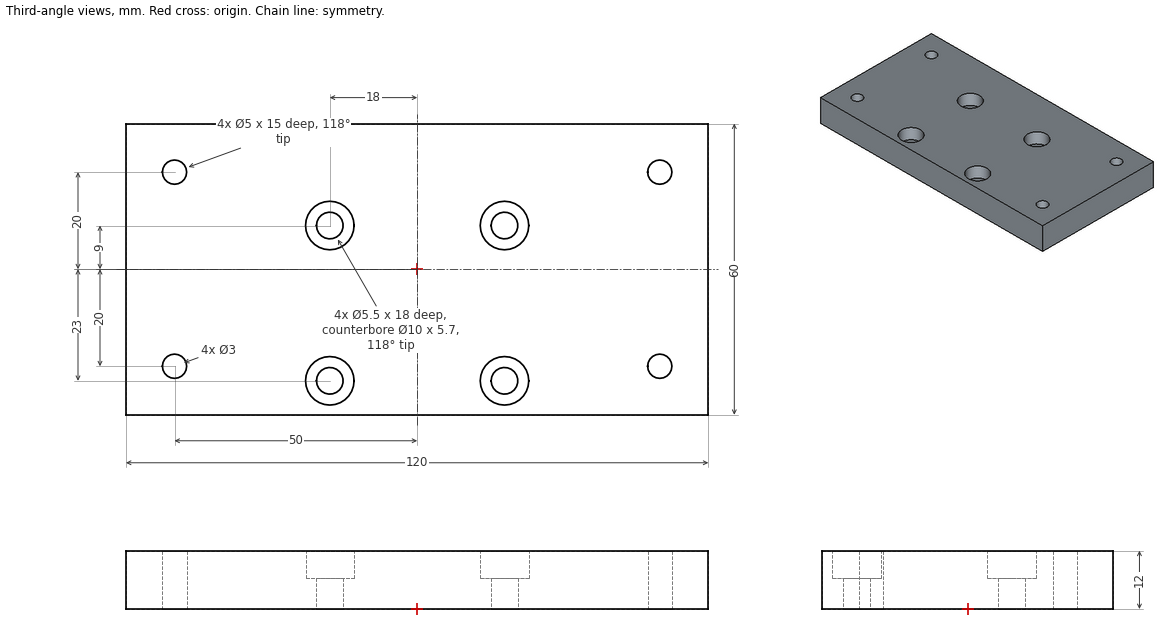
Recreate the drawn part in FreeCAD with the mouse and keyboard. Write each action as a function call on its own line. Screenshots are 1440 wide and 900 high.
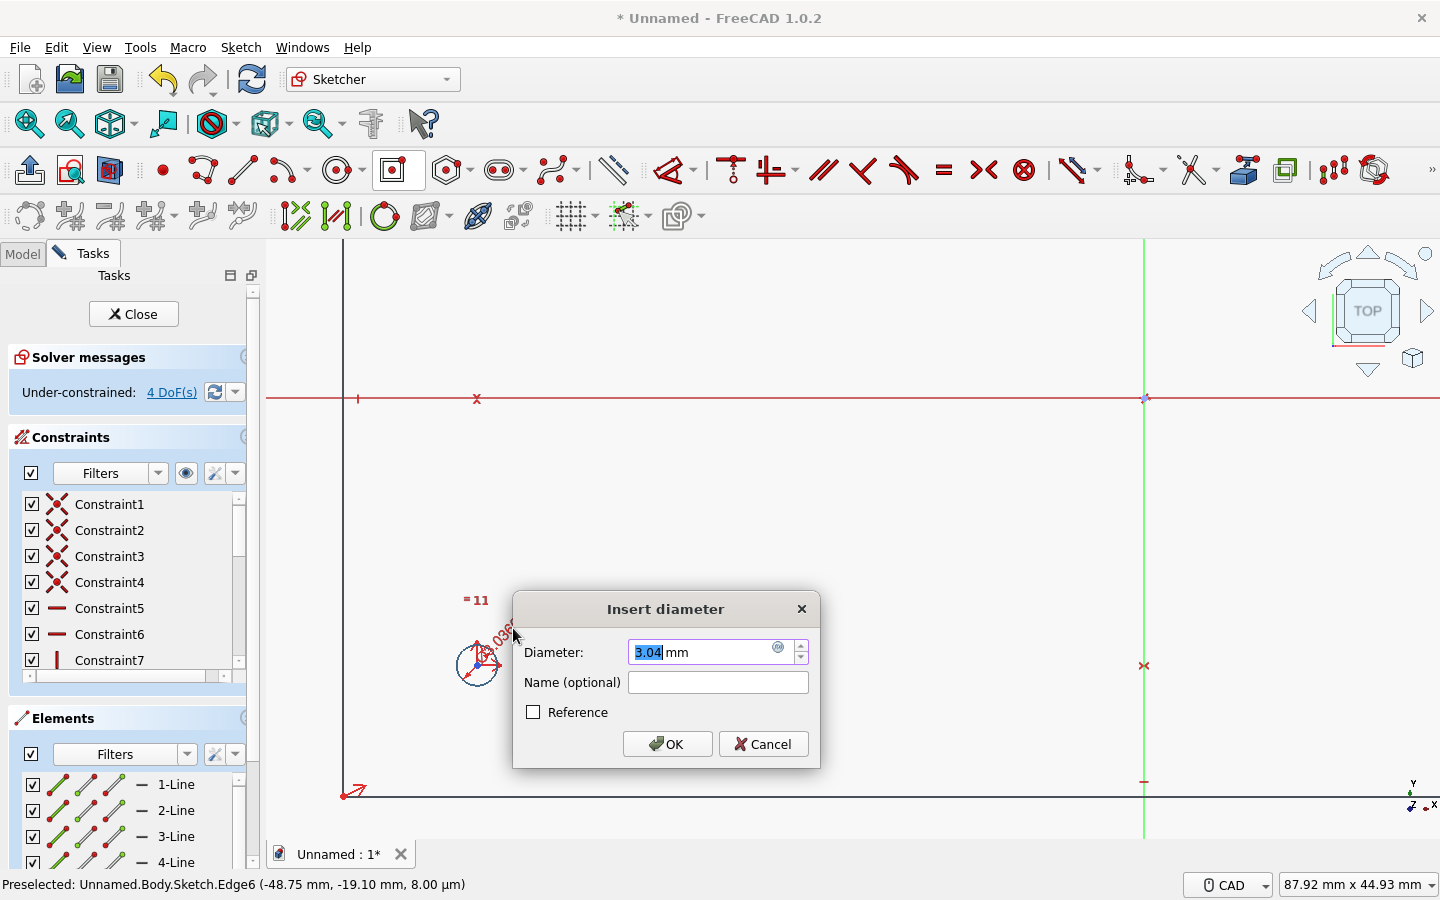
text(3)
key(Return)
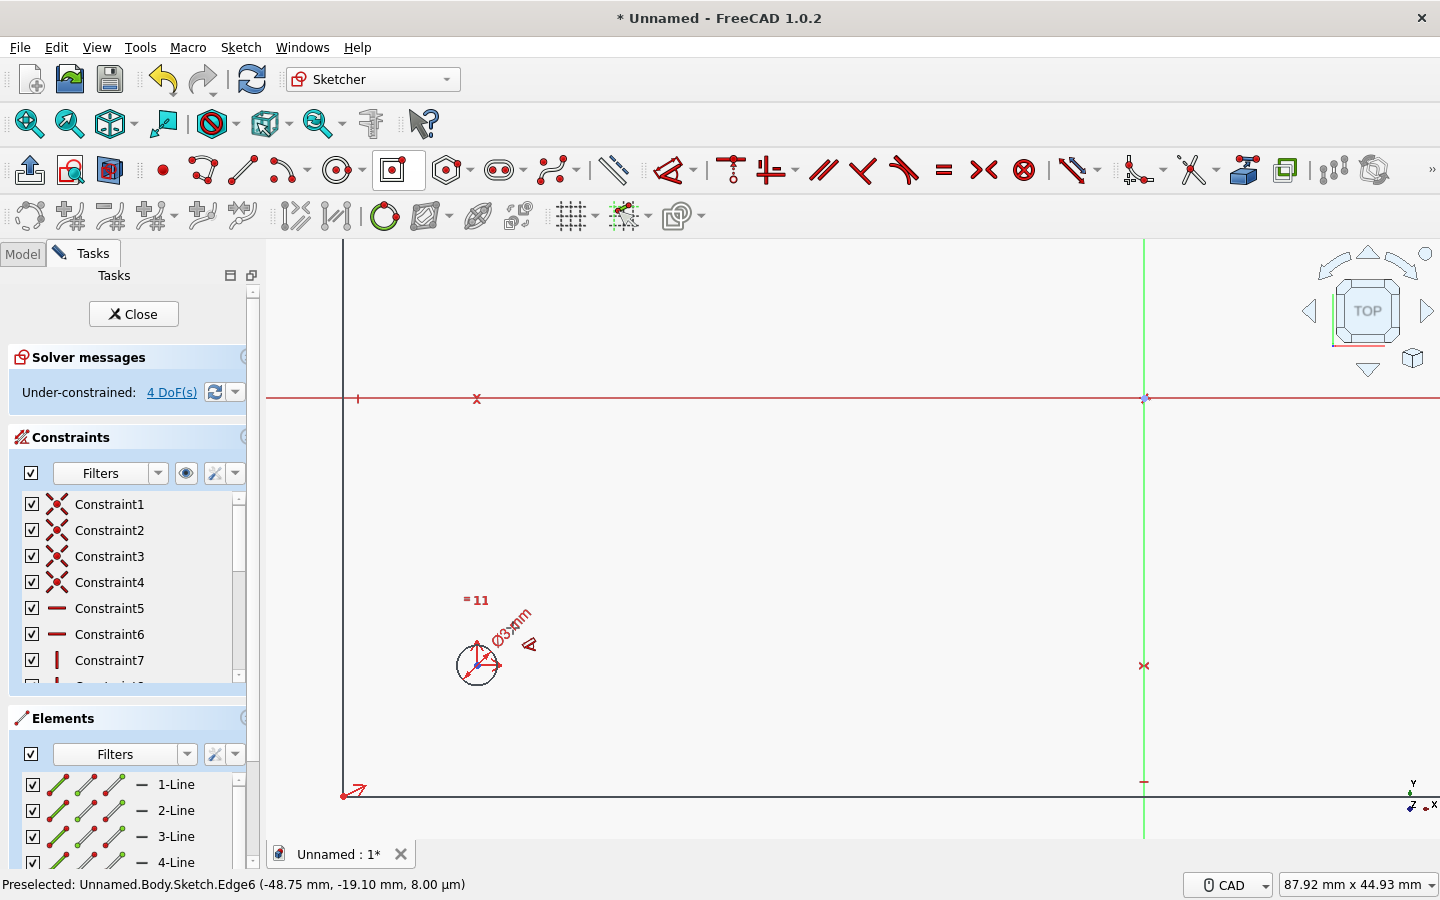
scroll(491, 654, down, 4)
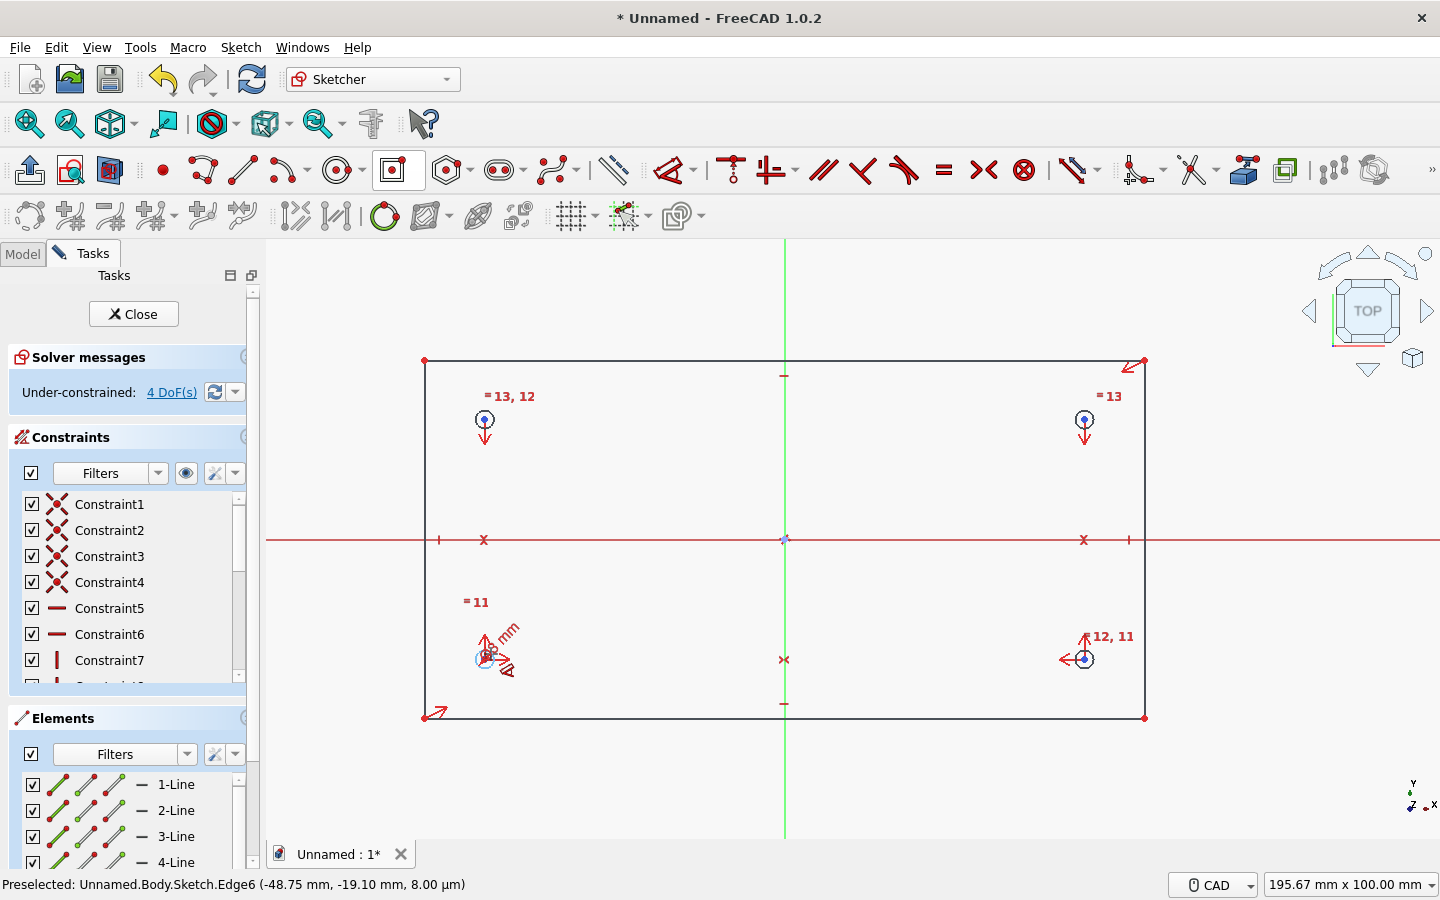
click(1145, 611)
click(1179, 457)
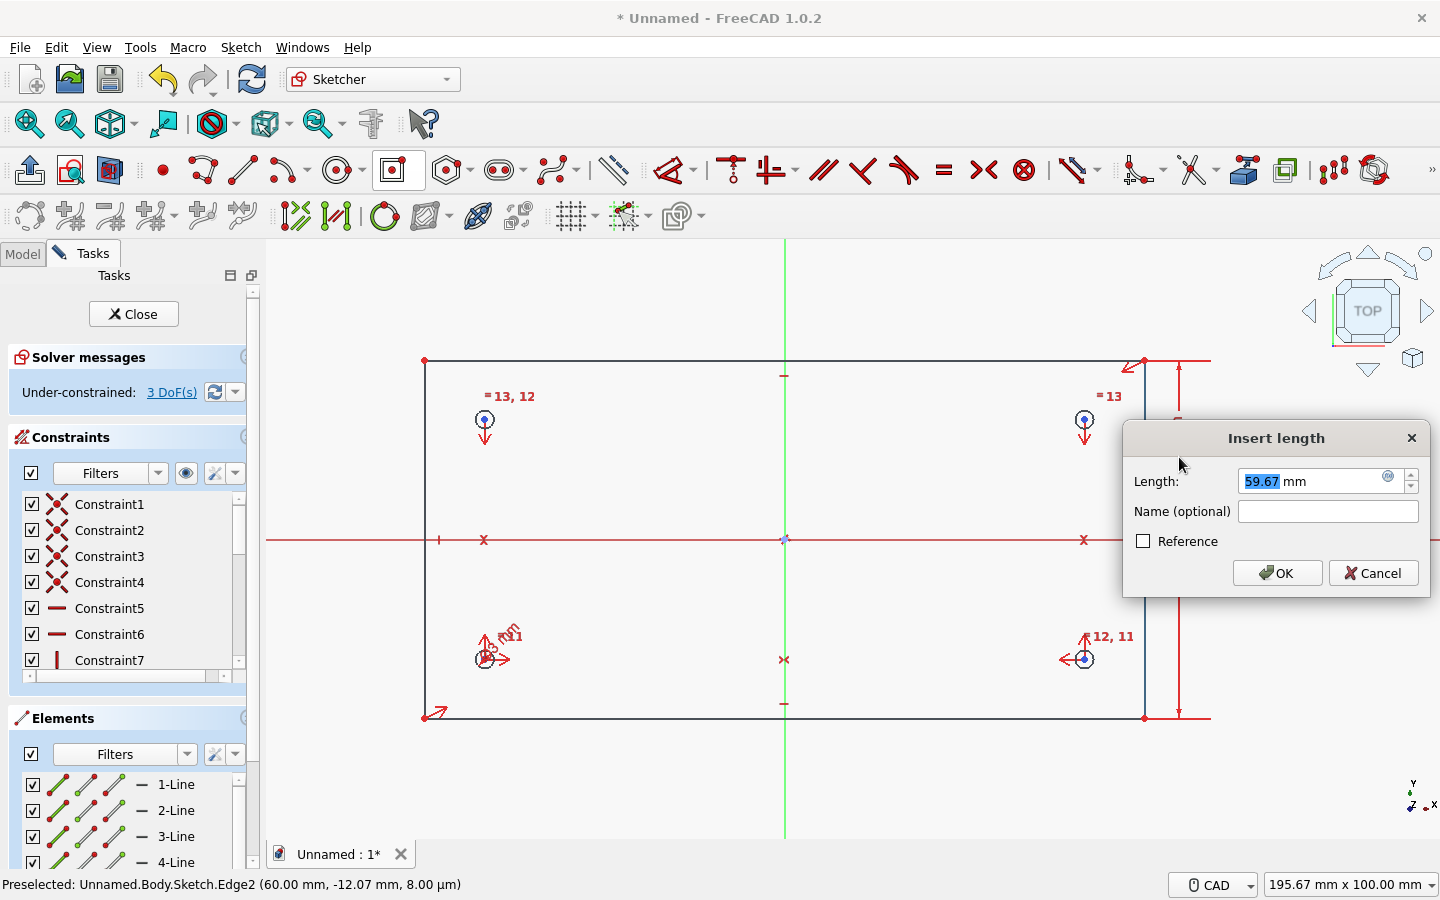
text(60)
key(Return)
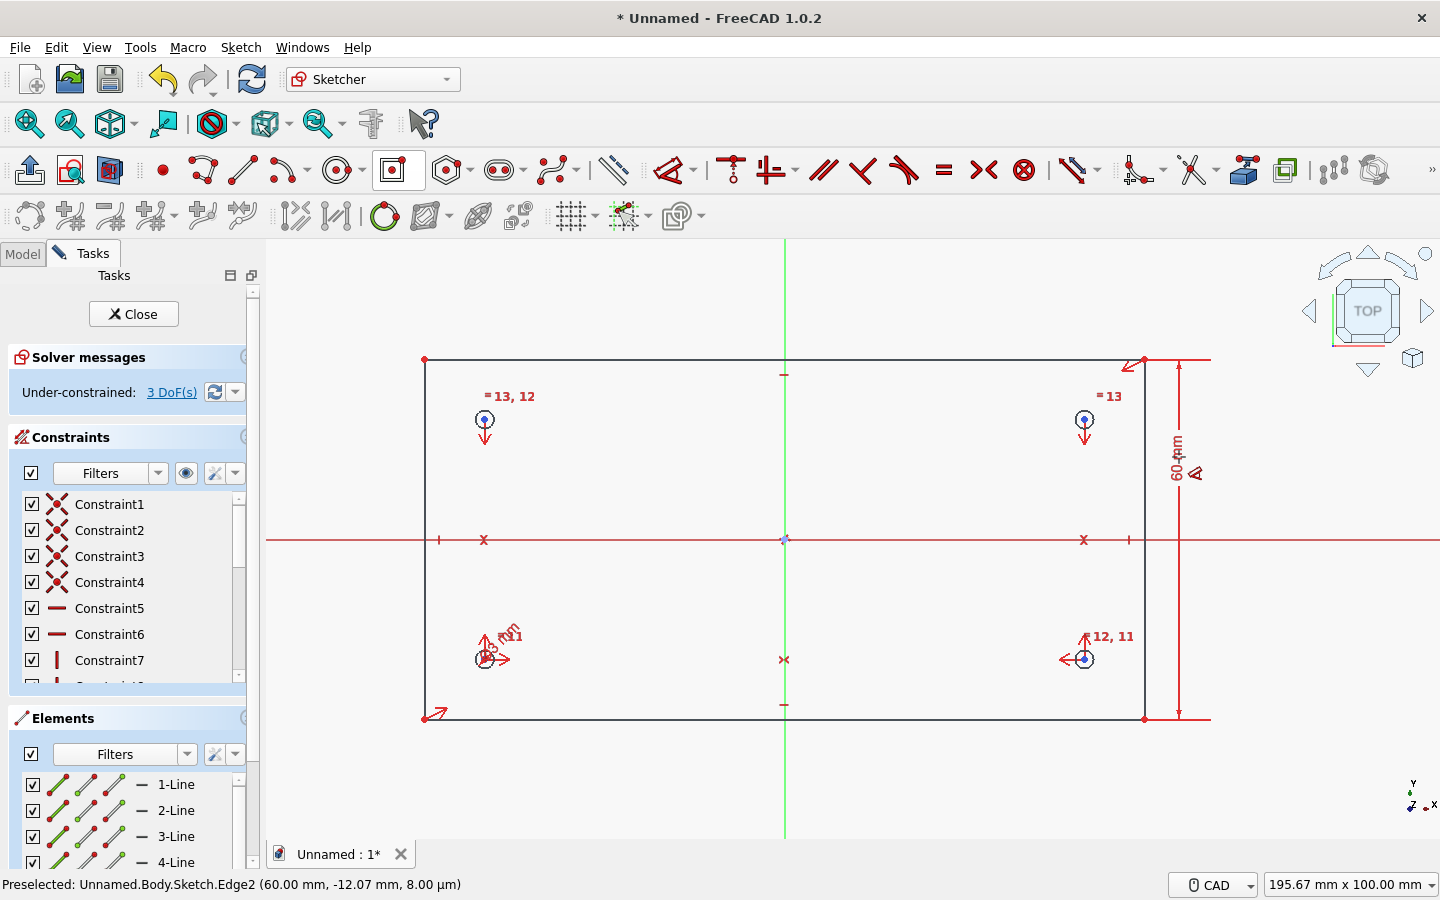
click(485, 660)
click(635, 694)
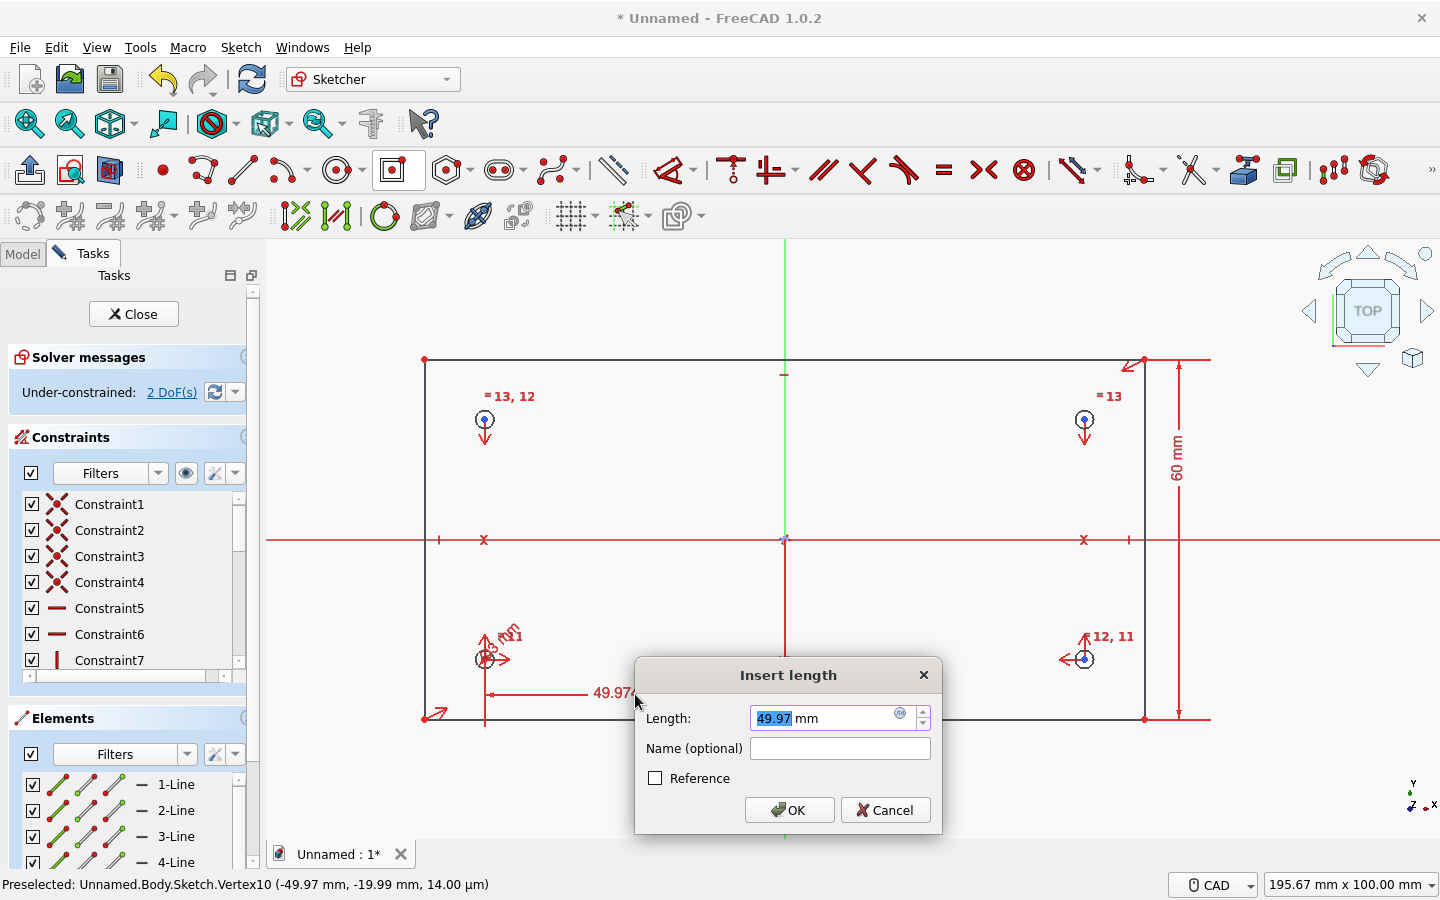
text(50)
key(Return)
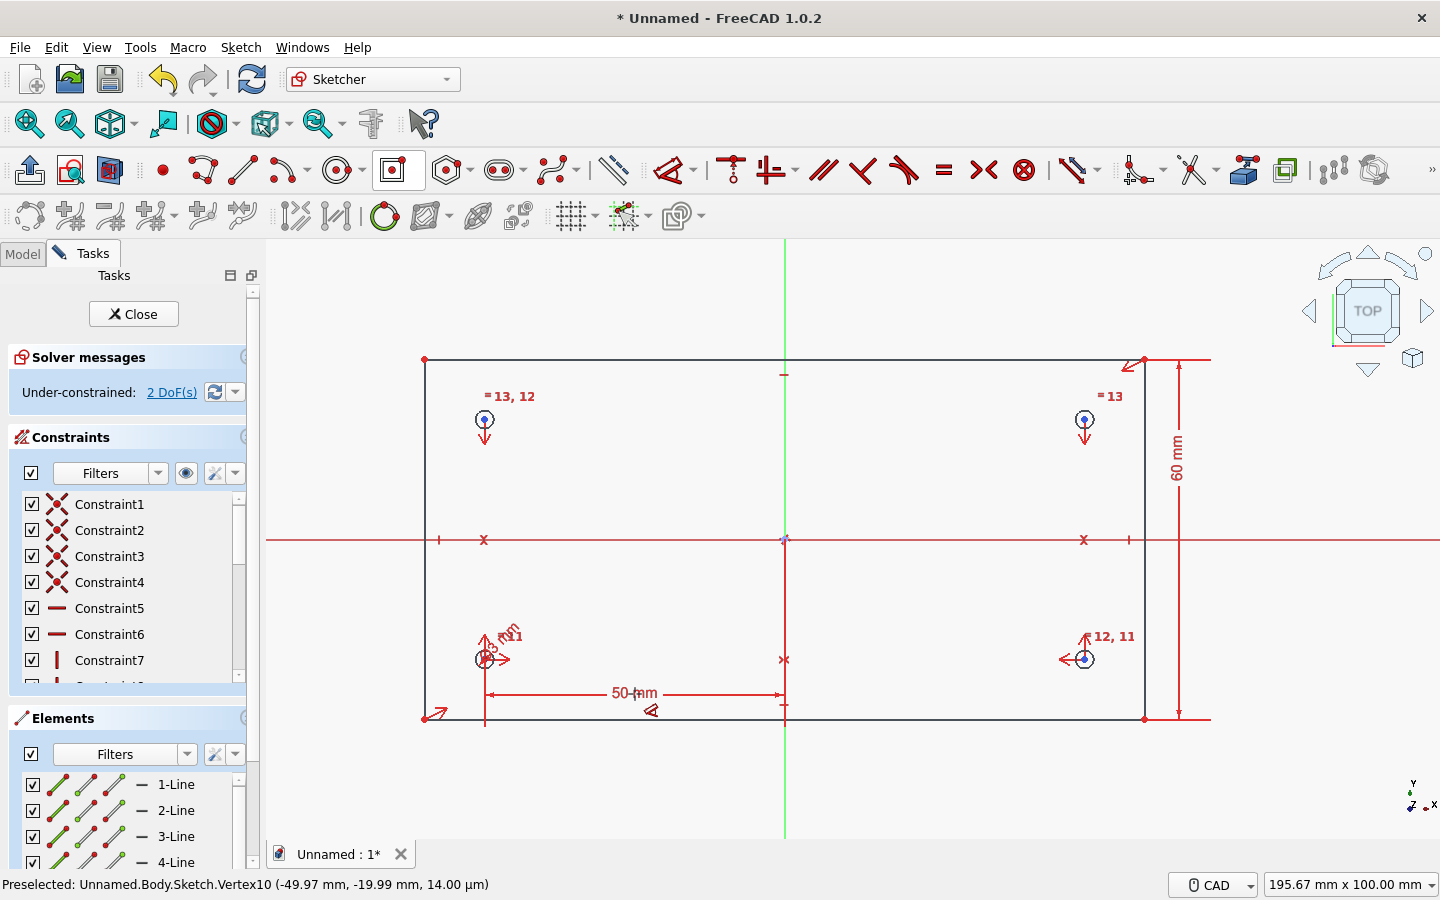
click(485, 660)
click(451, 600)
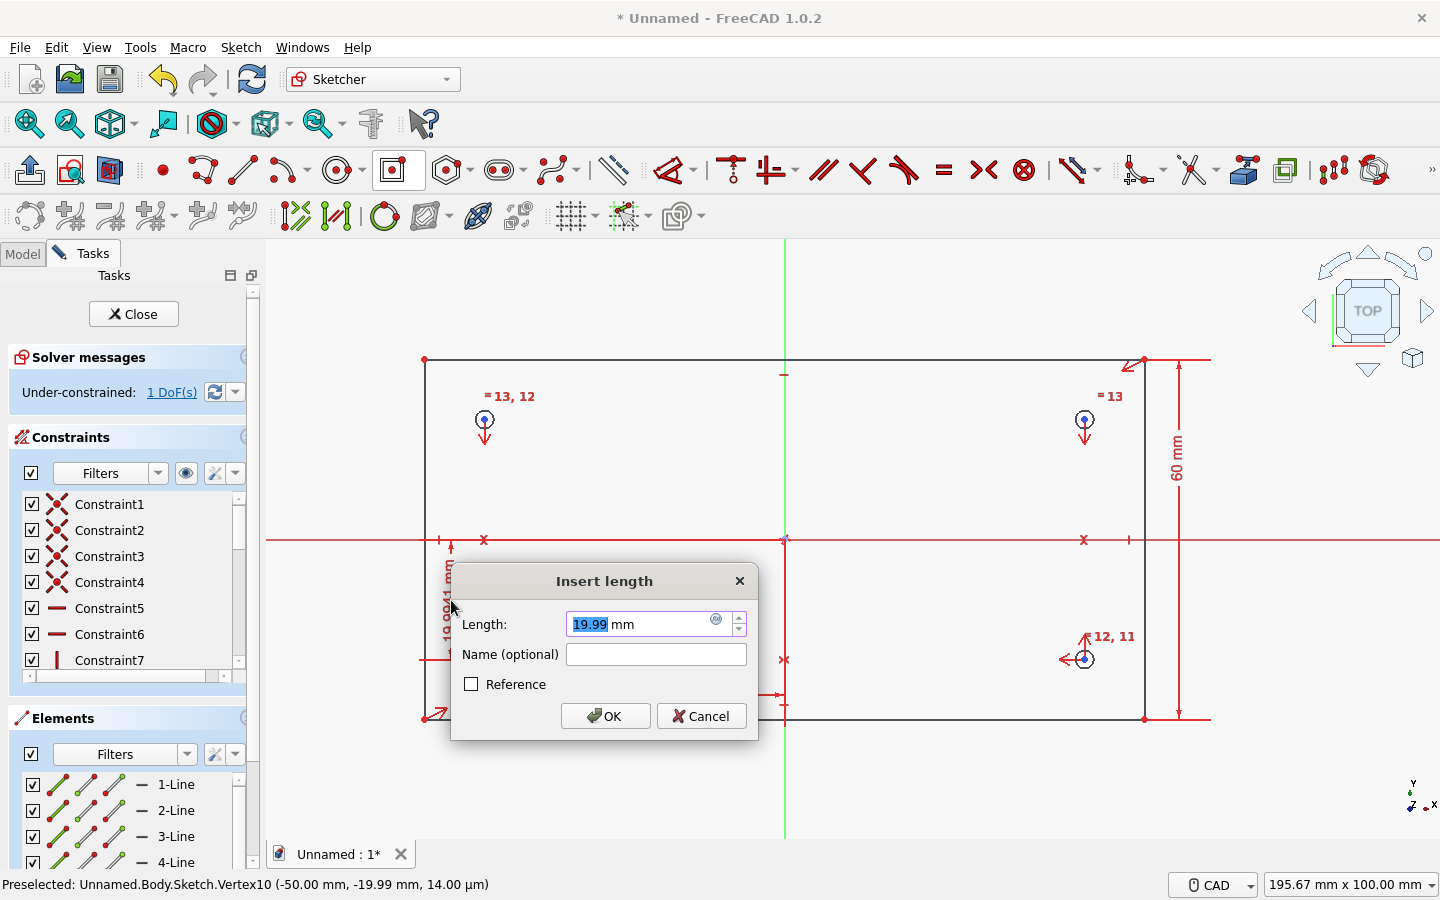
text(20)
key(Return)